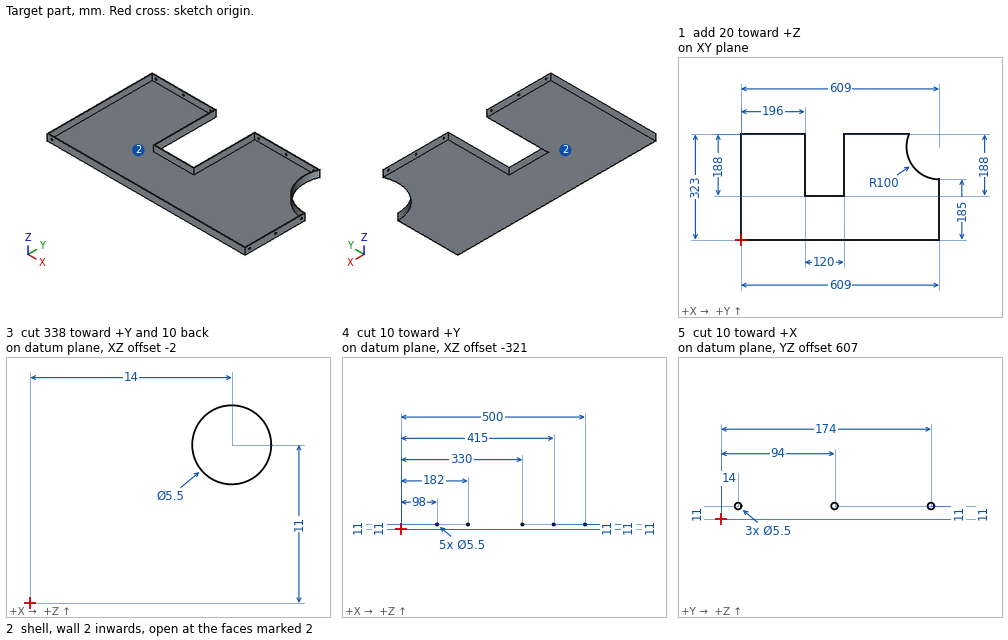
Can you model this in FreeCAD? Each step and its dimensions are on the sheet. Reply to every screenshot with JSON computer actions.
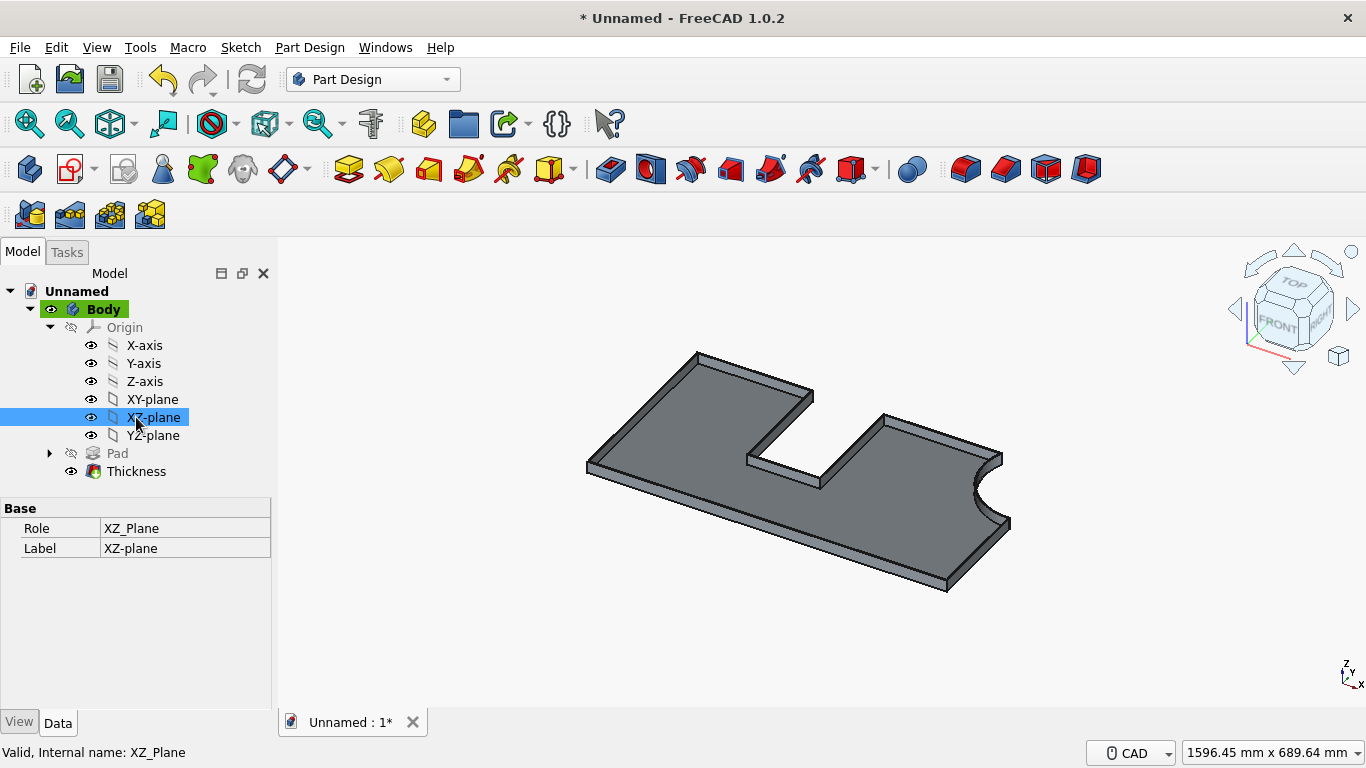
{"action": "left_click", "coordinate": [284, 170]}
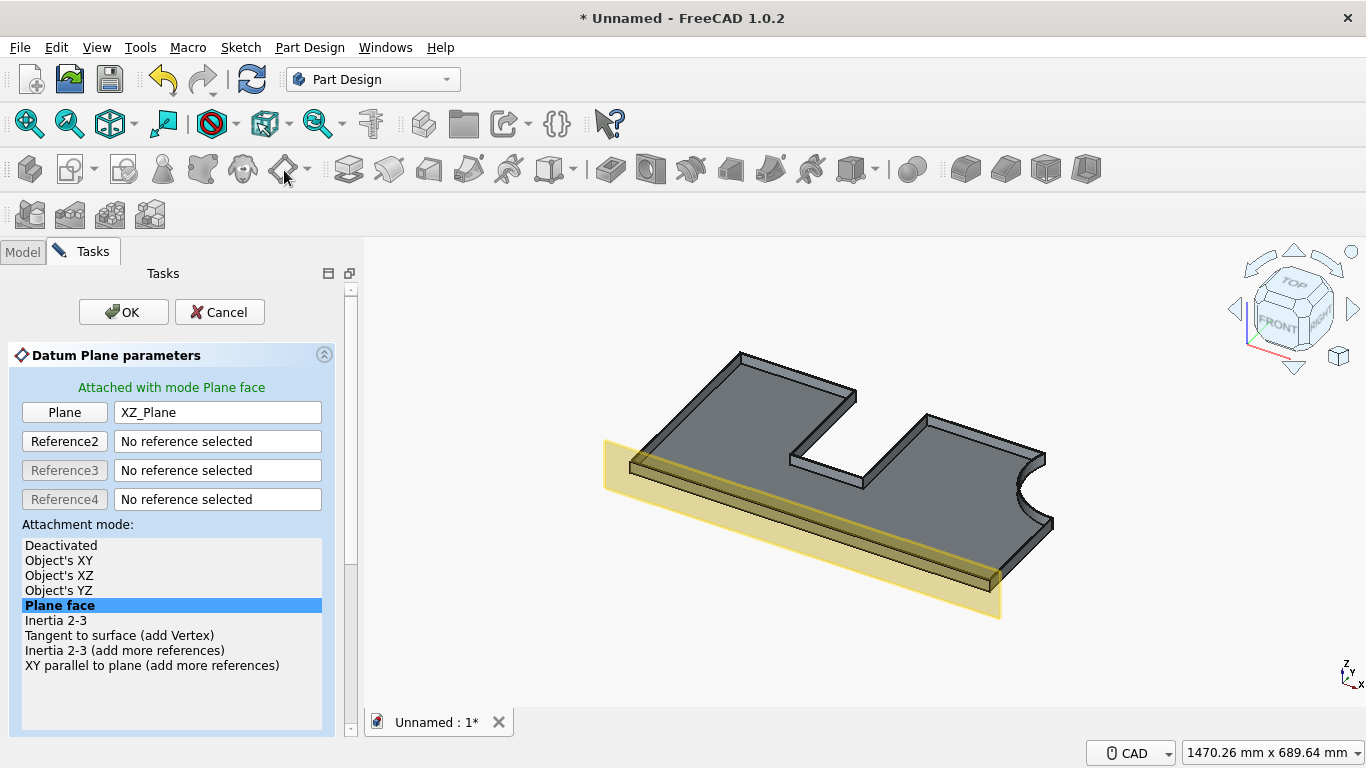
{"action": "scroll", "coordinate": [351, 510], "scroll_direction": "down", "scroll_amount": 3}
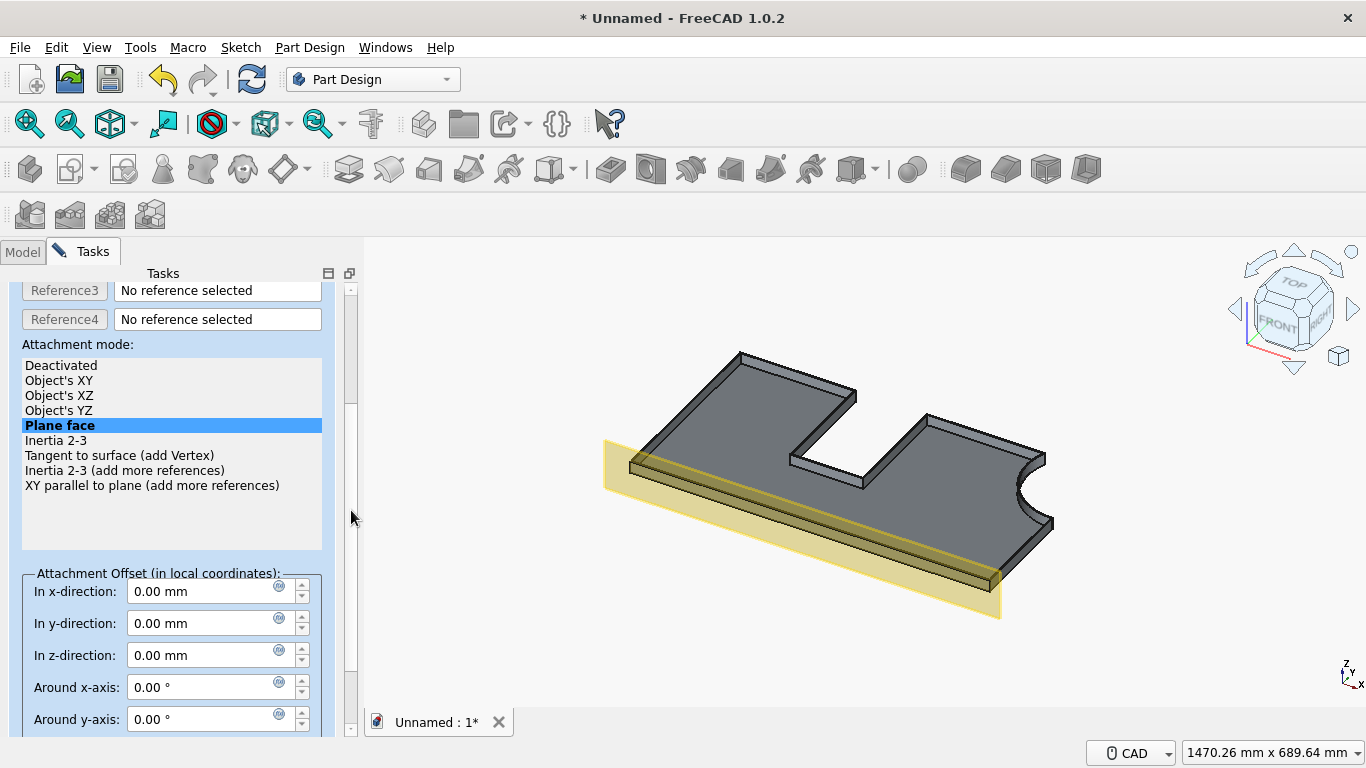
{"action": "triple_click", "coordinate": [210, 655]}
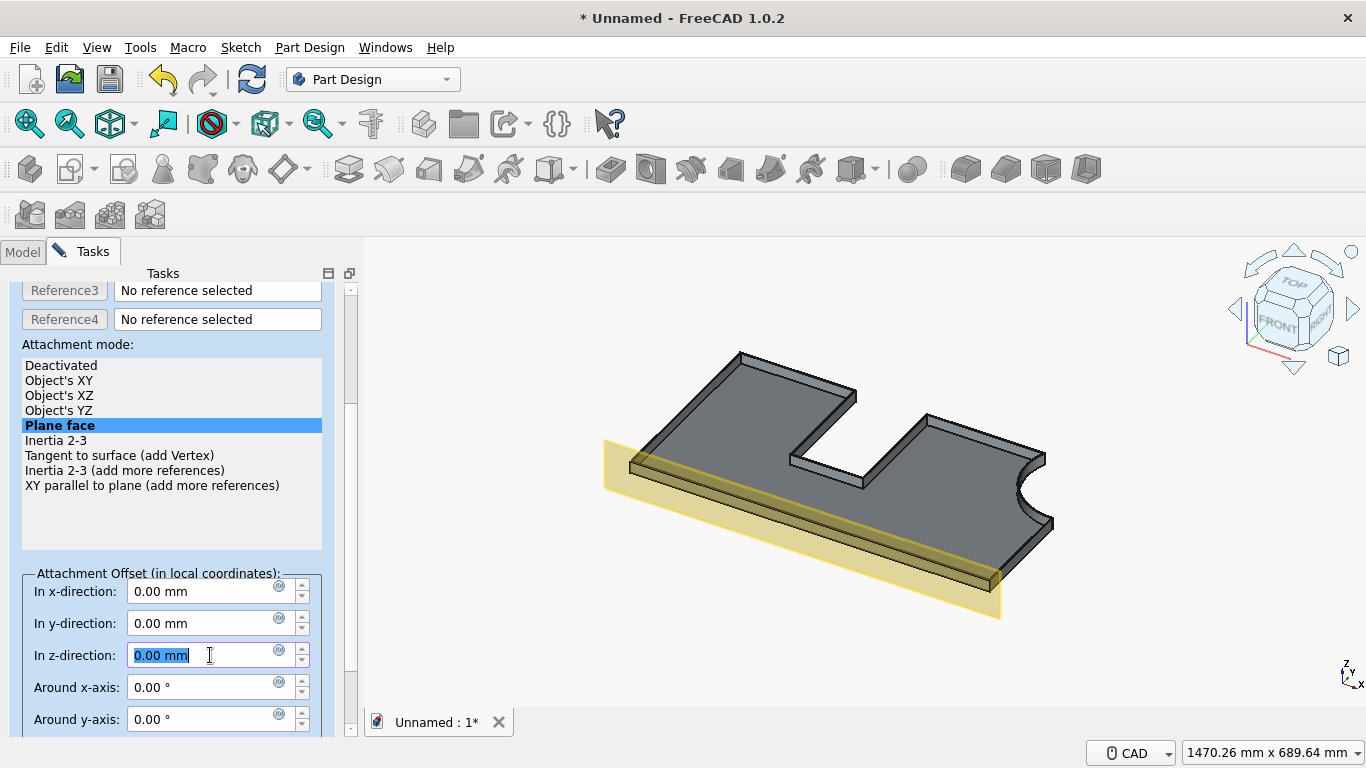
{"action": "type", "text": "-2"}
{"action": "key", "text": "Tab"}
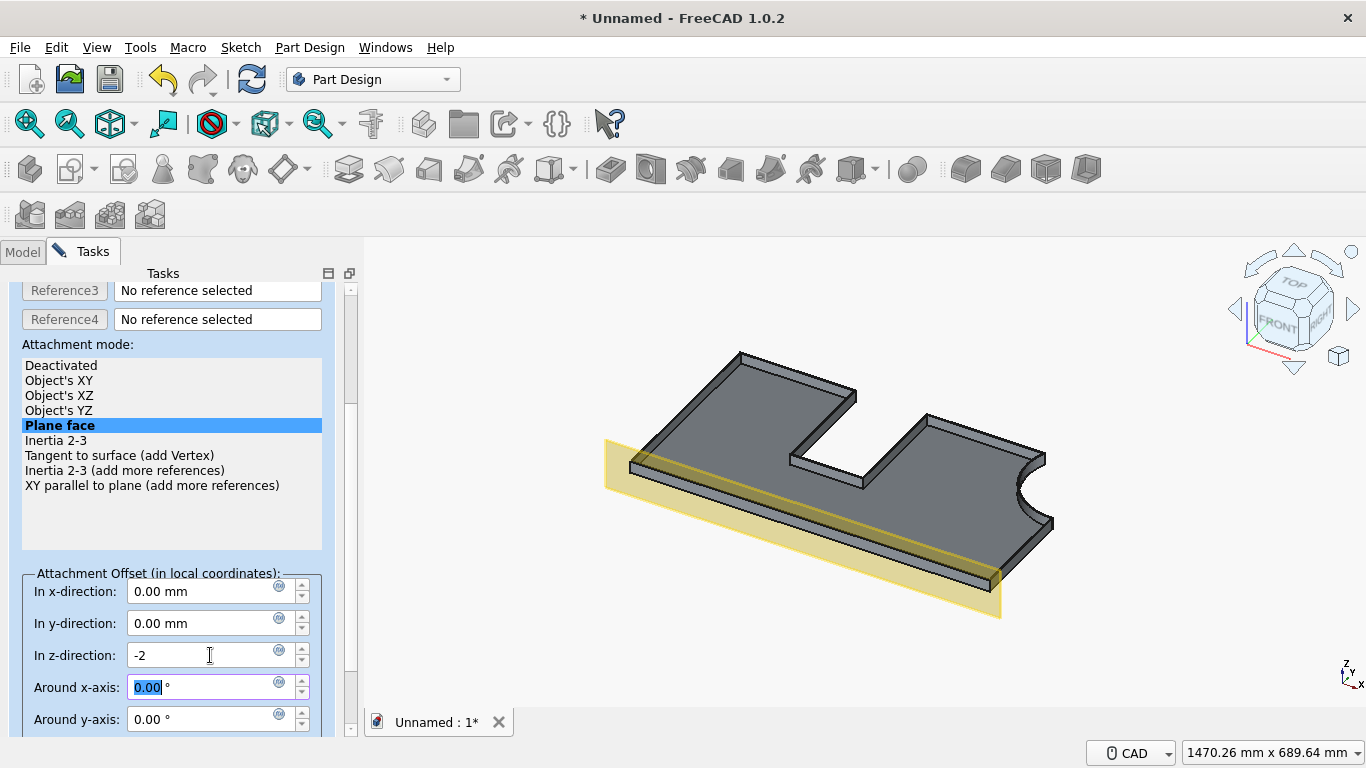
{"action": "scroll", "coordinate": [351, 510], "scroll_direction": "up", "scroll_amount": 4}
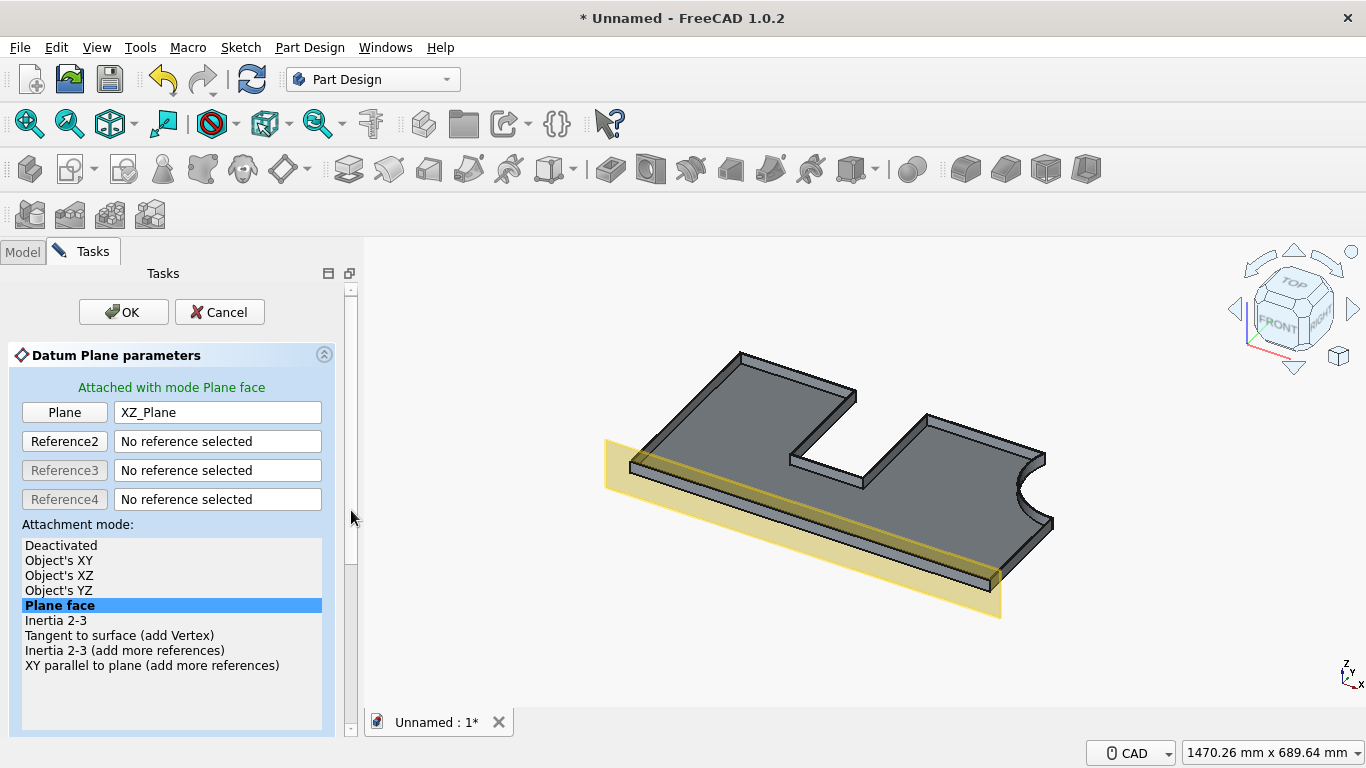
{"action": "left_click", "coordinate": [124, 312]}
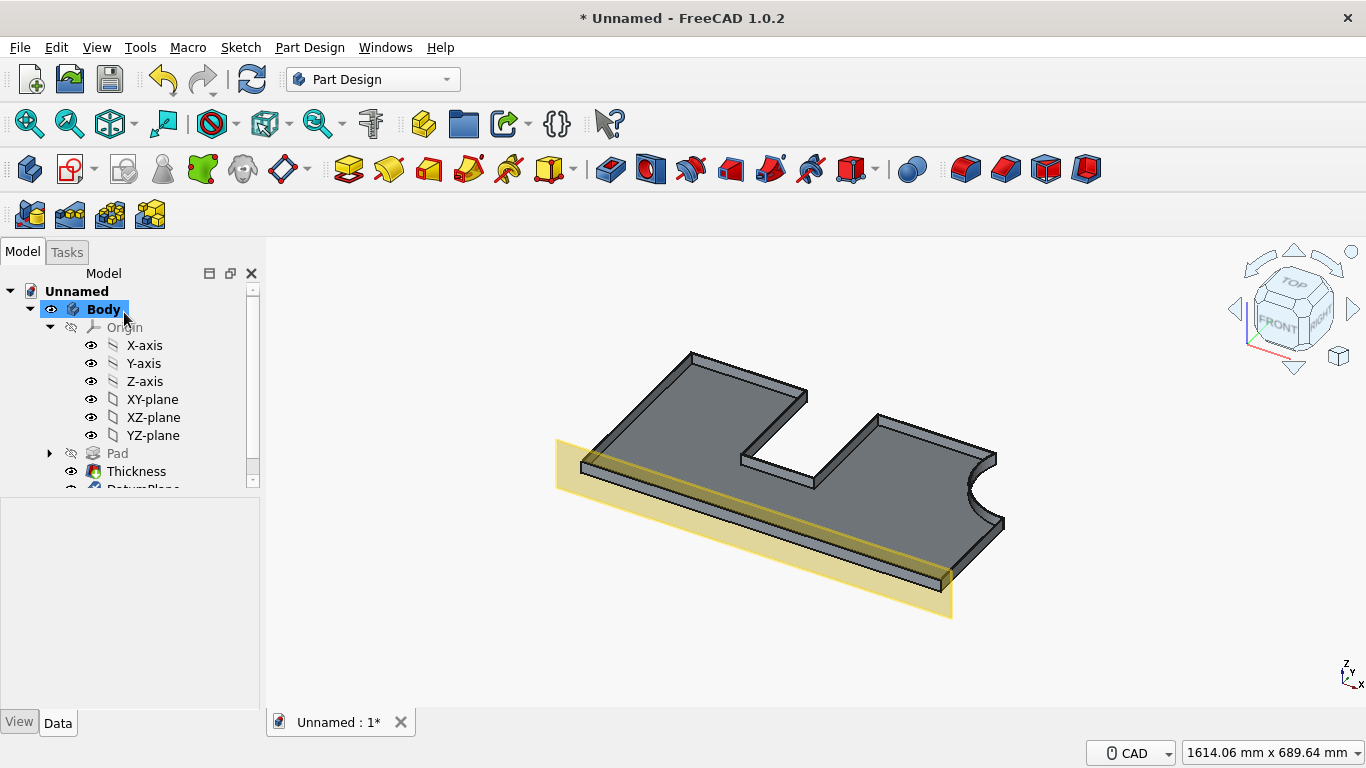
{"action": "scroll", "coordinate": [100, 377], "scroll_direction": "down", "scroll_amount": 3}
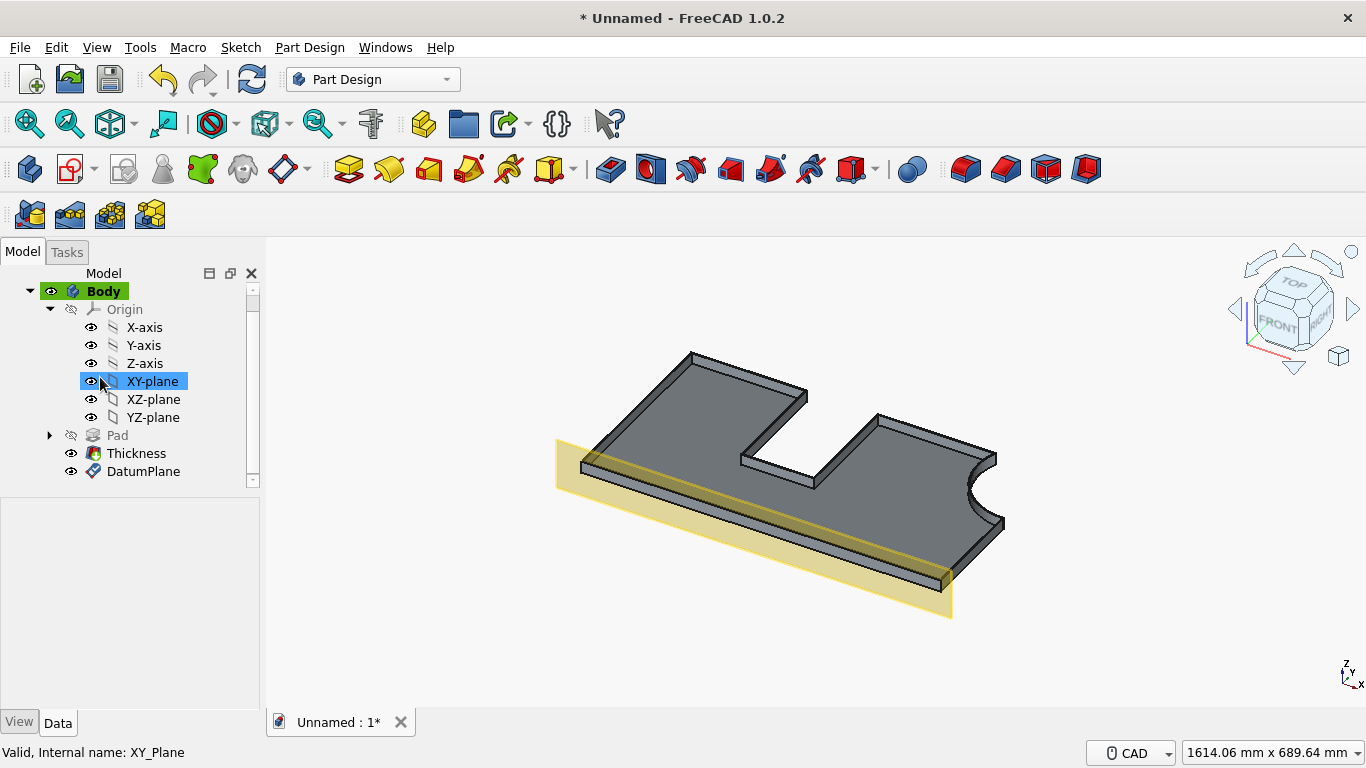
{"action": "left_click", "coordinate": [116, 471]}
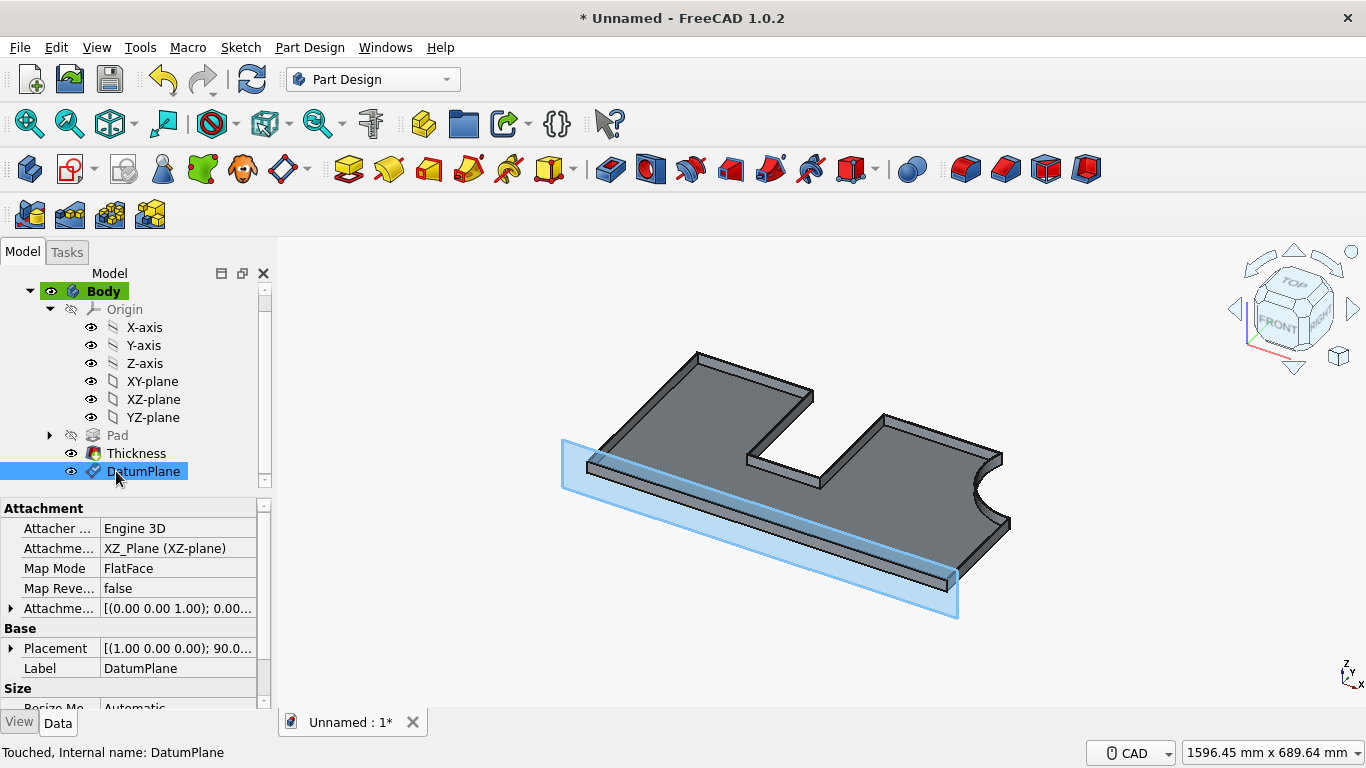
{"action": "left_click", "coordinate": [70, 170]}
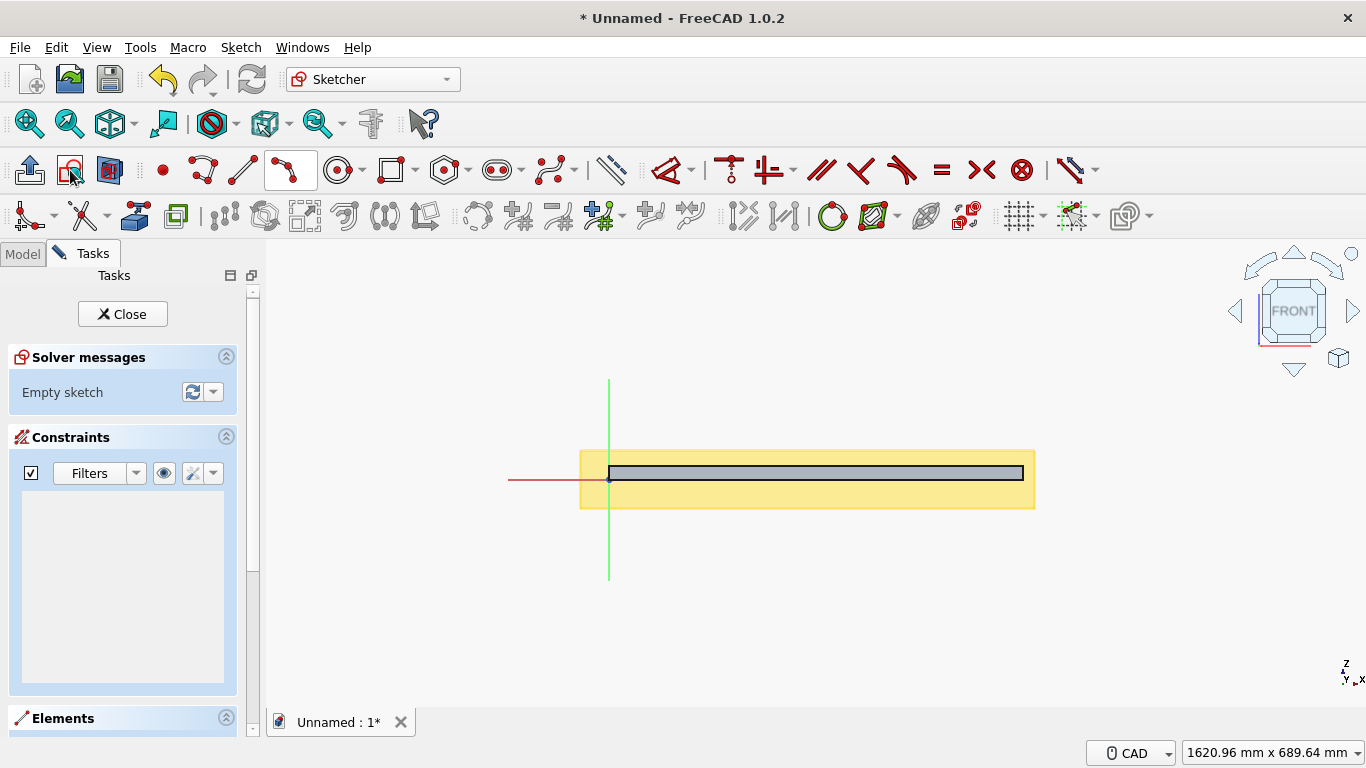
{"action": "left_click", "coordinate": [110, 170]}